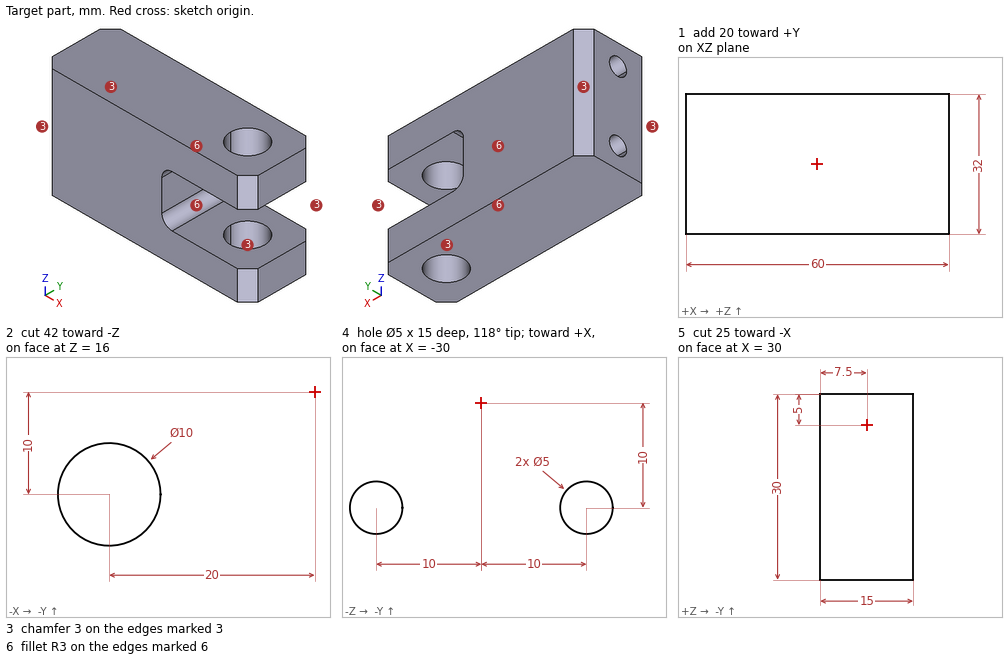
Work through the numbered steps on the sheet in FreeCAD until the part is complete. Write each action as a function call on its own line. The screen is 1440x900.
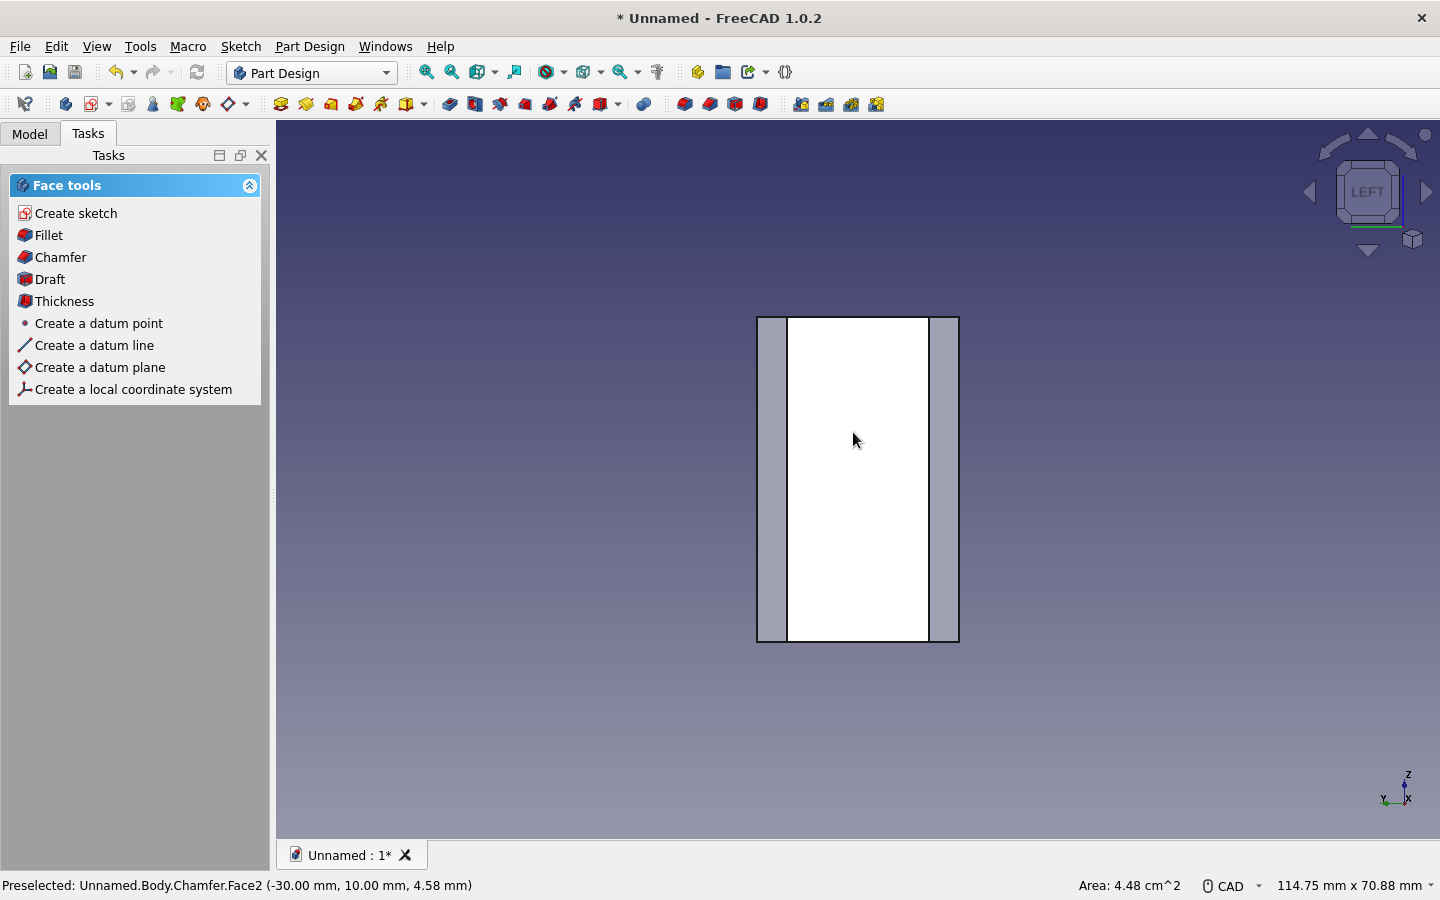
click(90, 104)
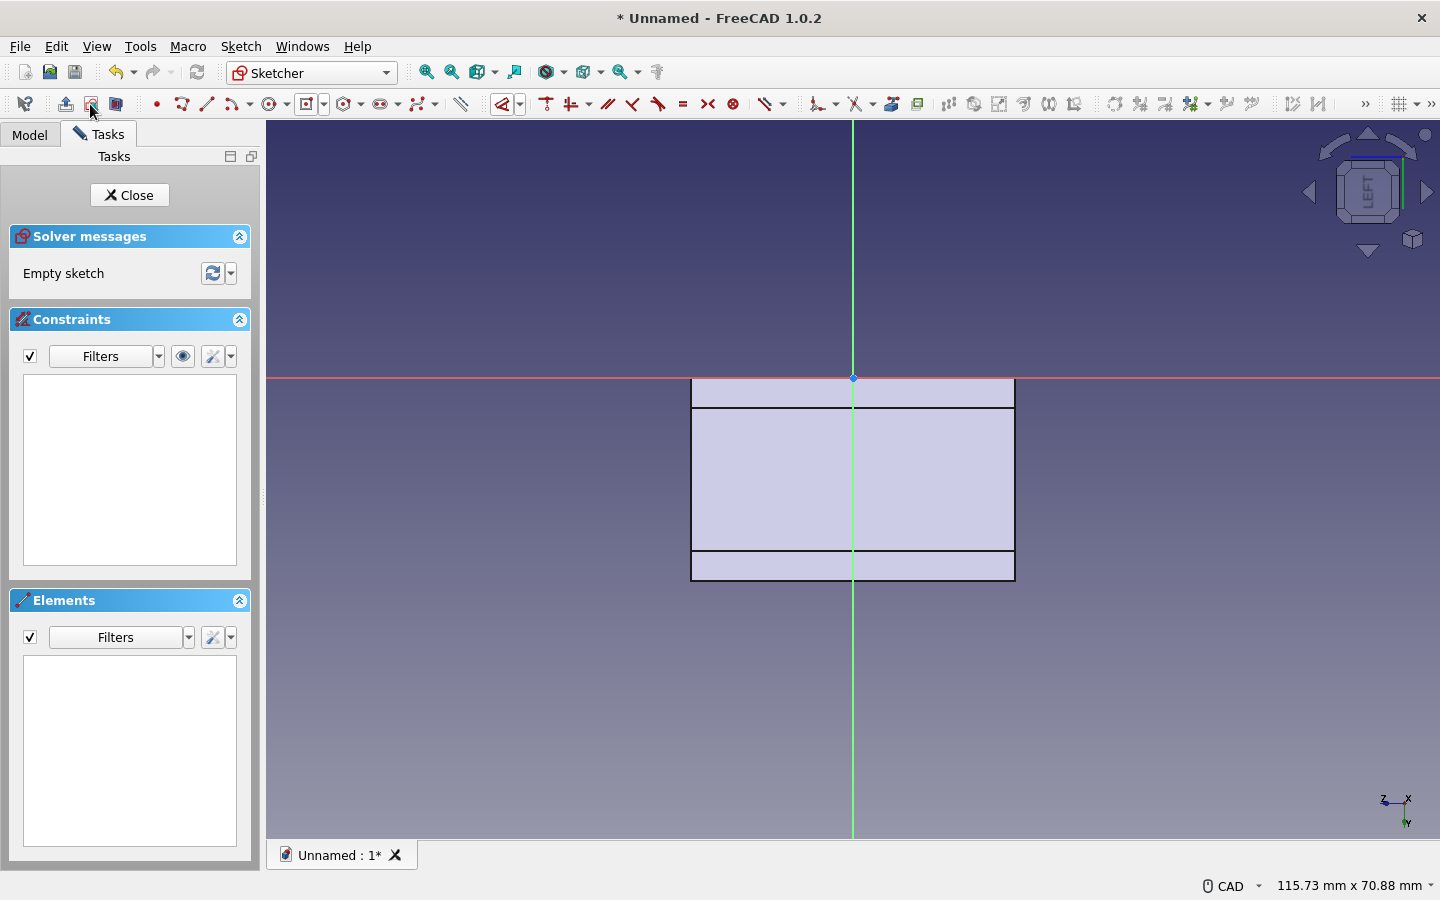
scroll(893, 419, up, 5)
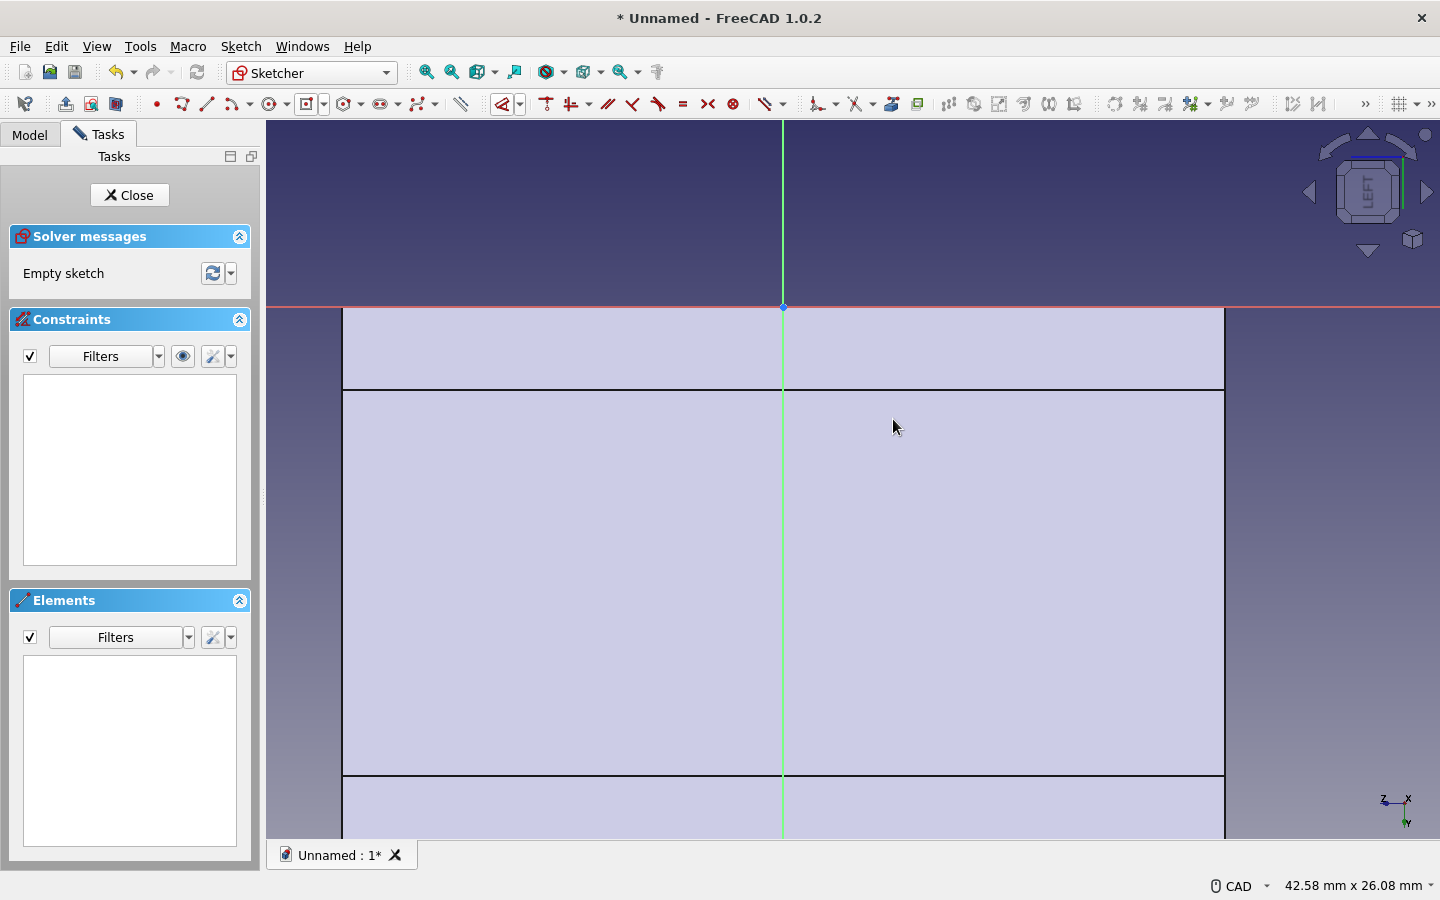
click(268, 104)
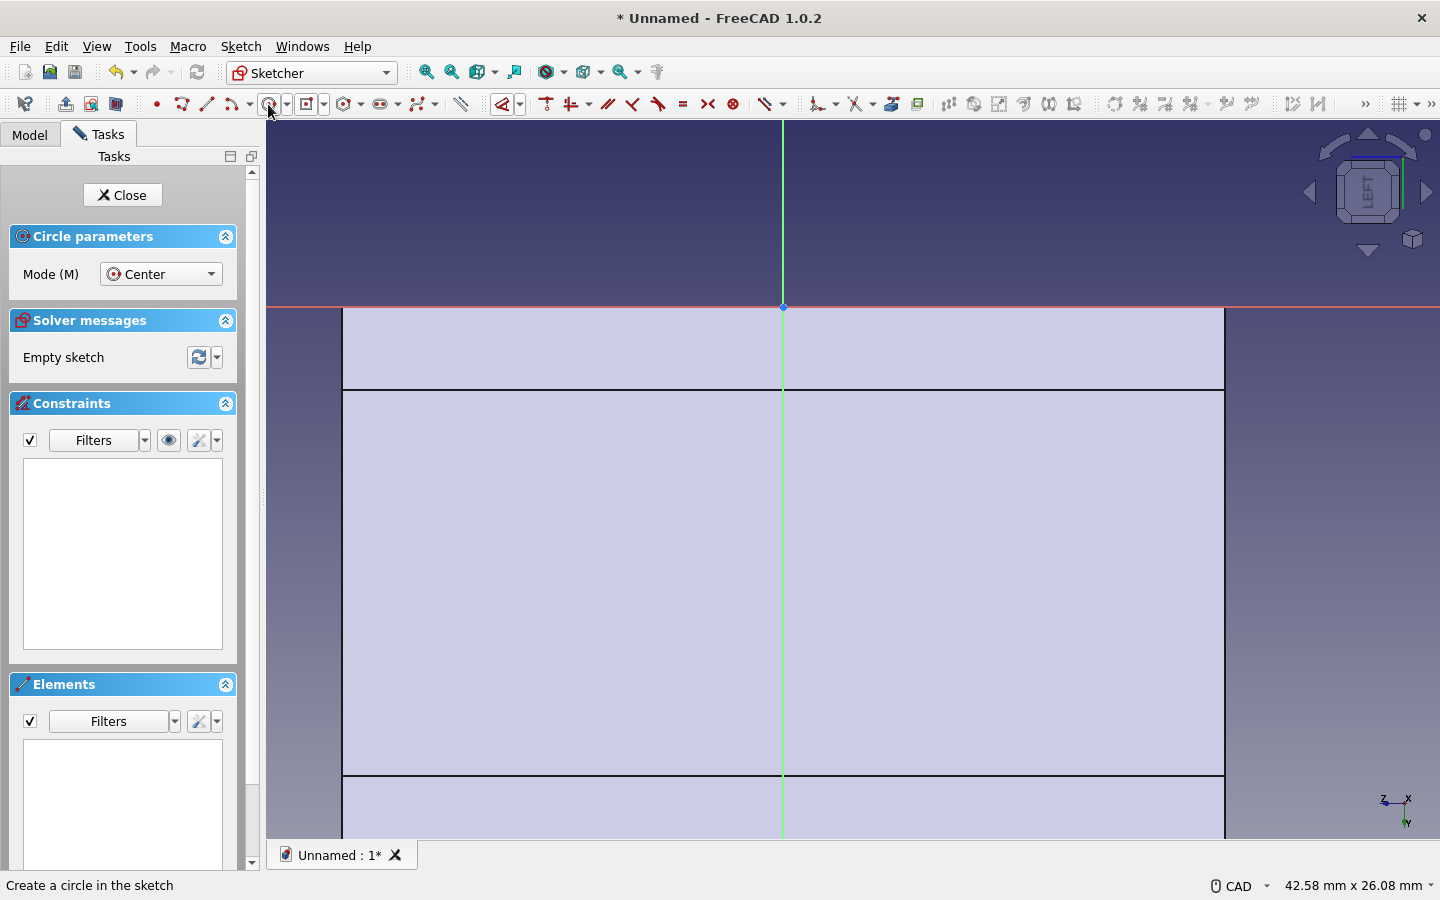
click(1059, 583)
click(1108, 534)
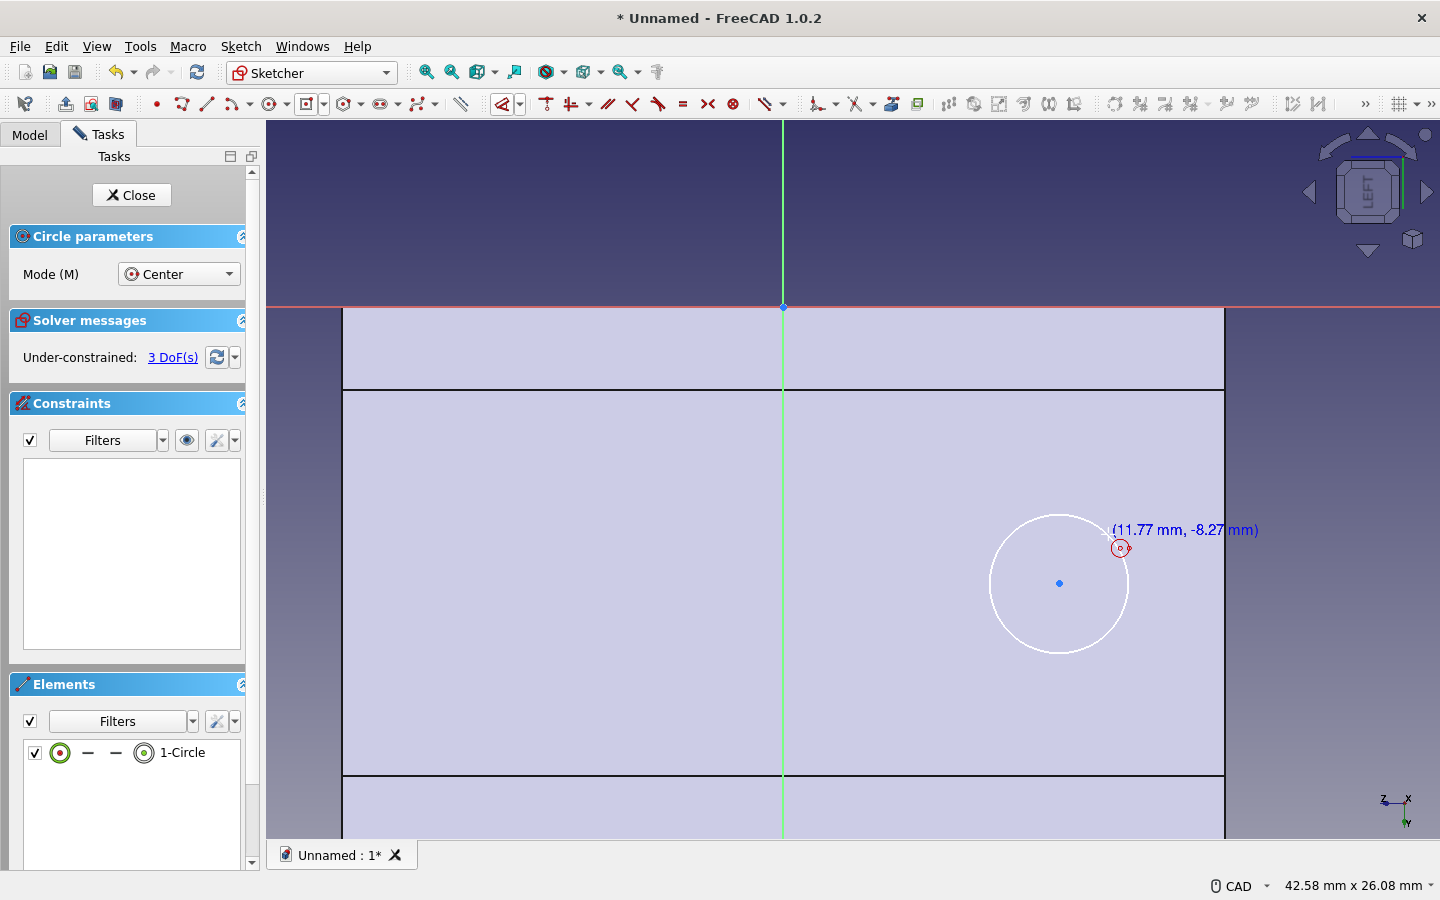
click(508, 583)
click(556, 534)
key(Escape)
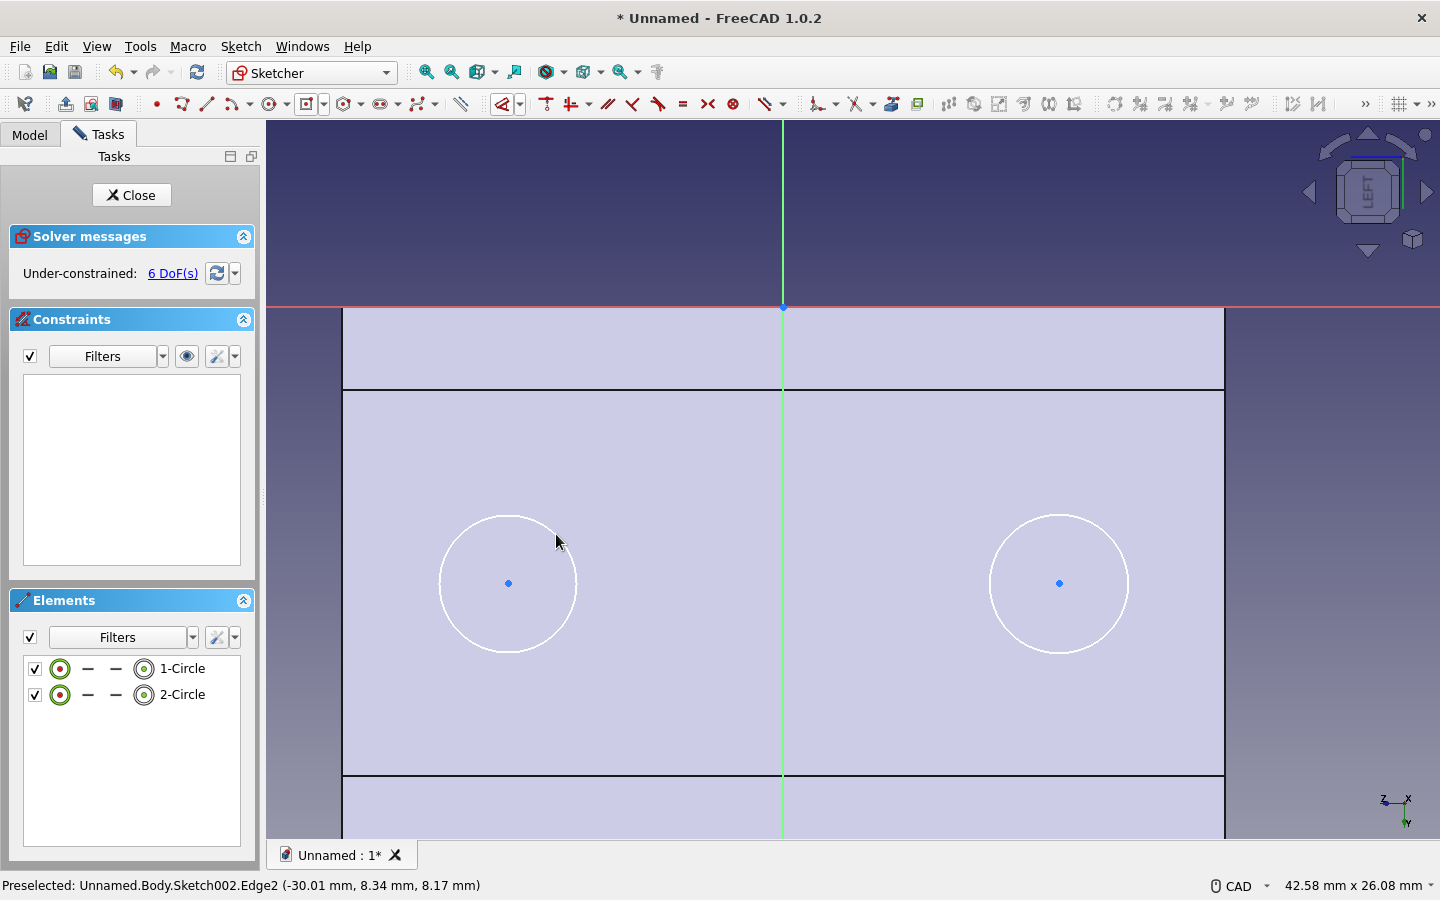
click(1108, 535)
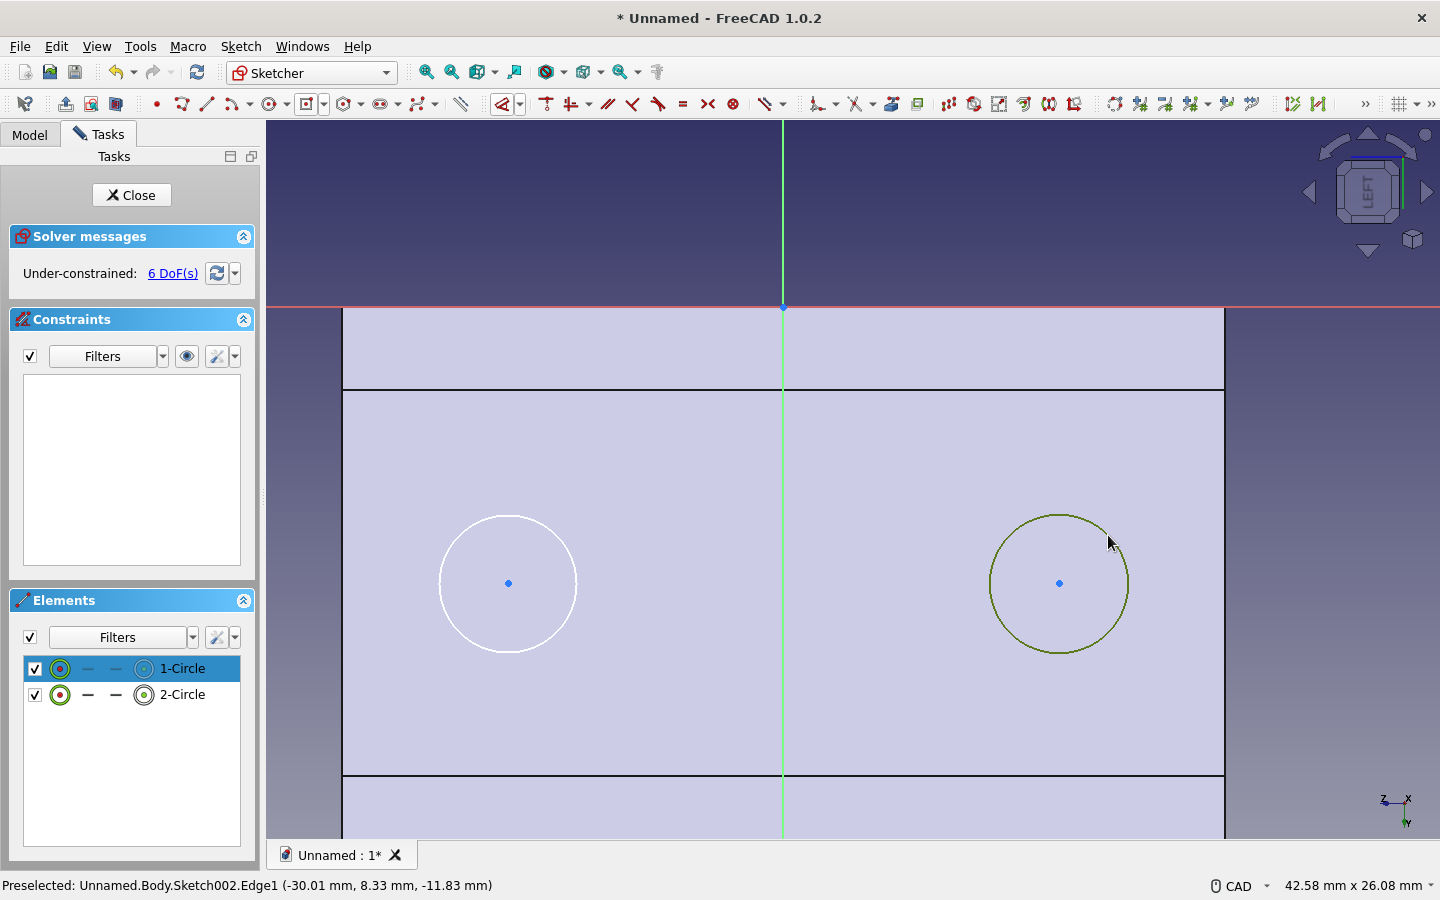
click(556, 535)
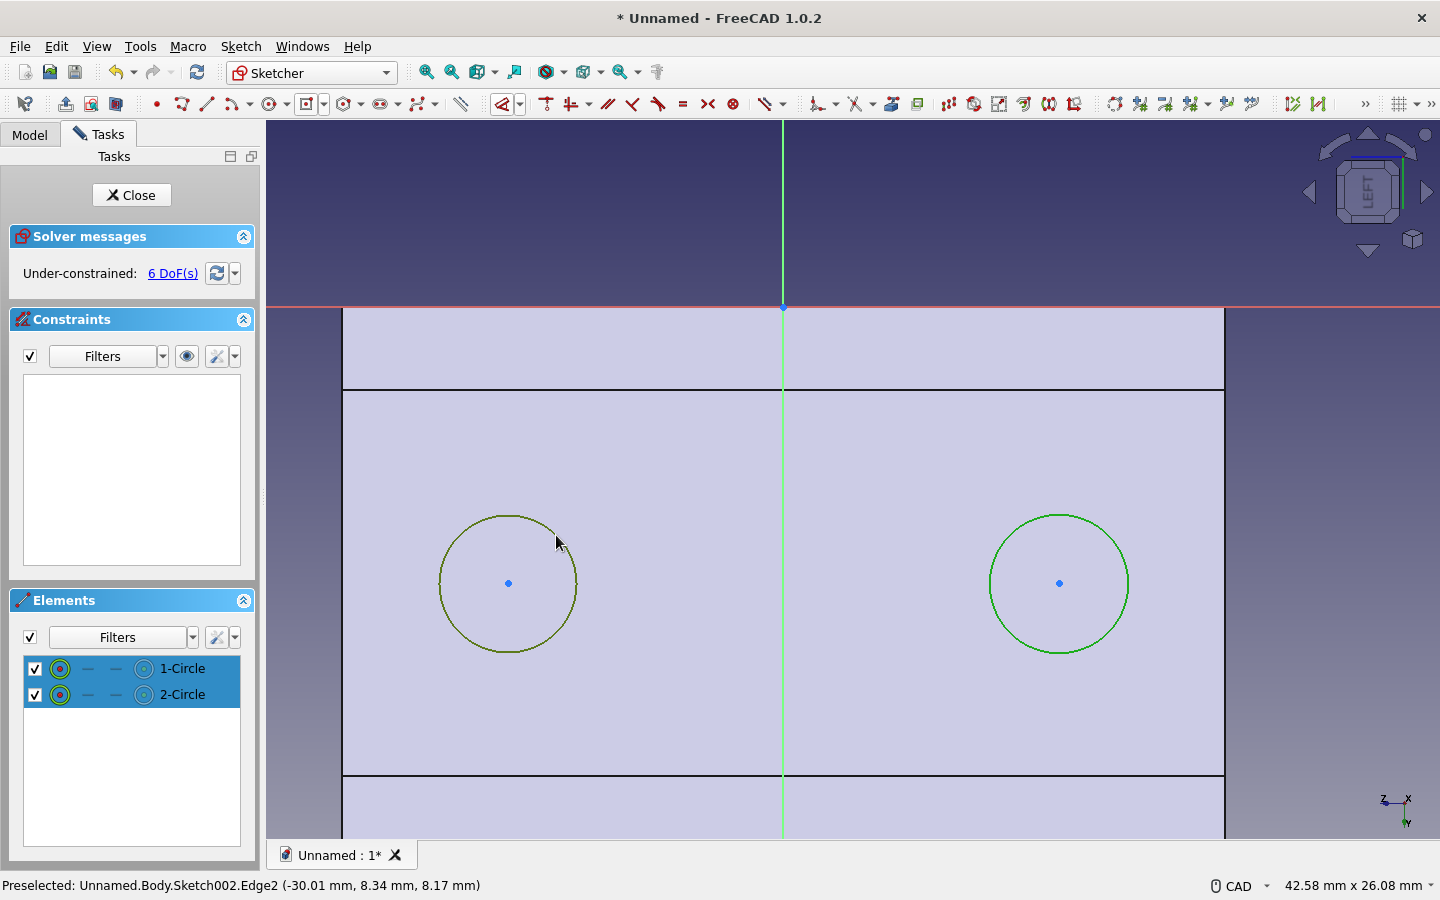
click(683, 104)